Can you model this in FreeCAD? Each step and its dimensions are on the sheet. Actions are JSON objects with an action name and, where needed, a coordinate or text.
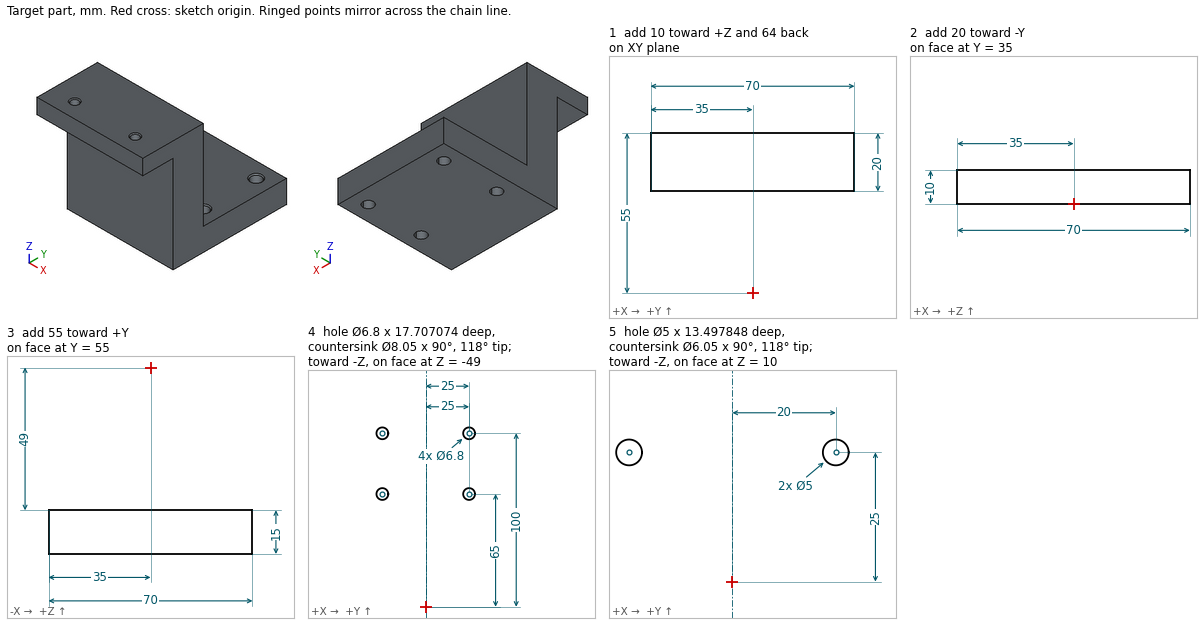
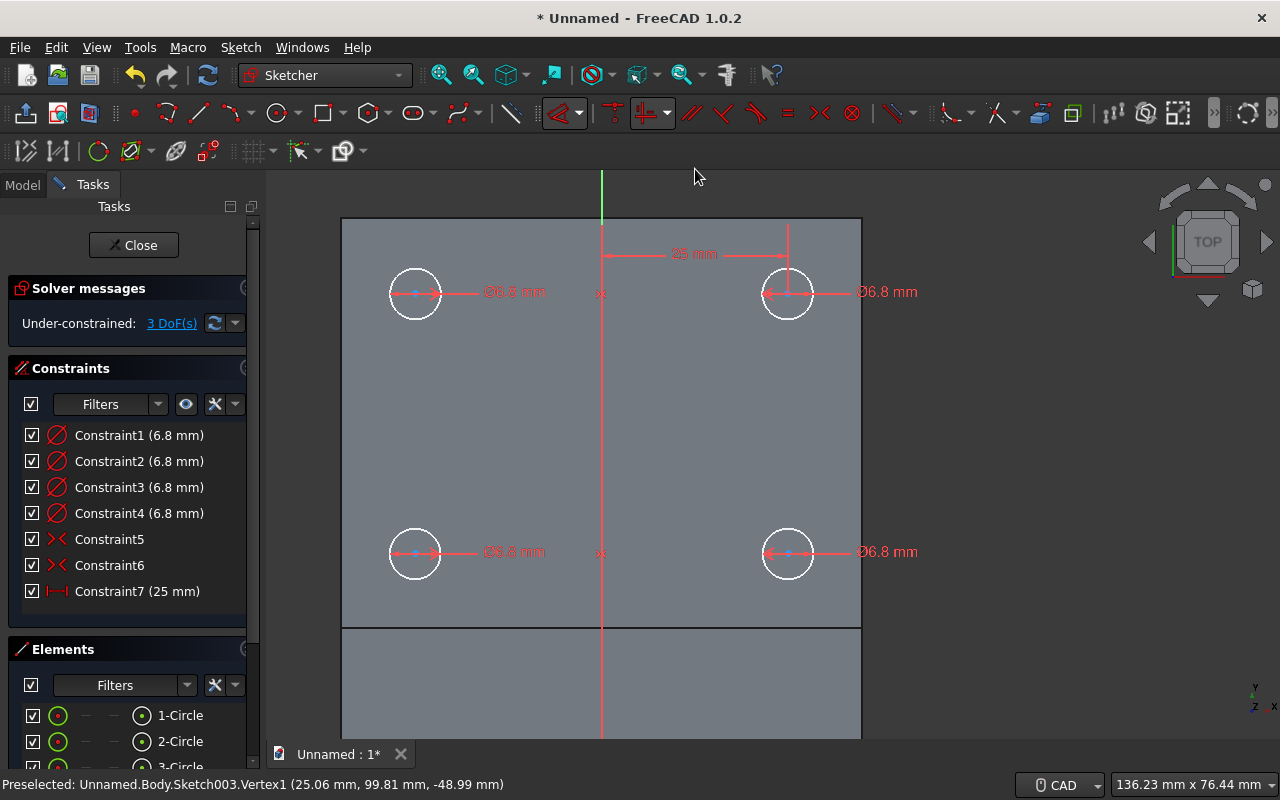
{"action": "left_click", "coordinate": [788, 554]}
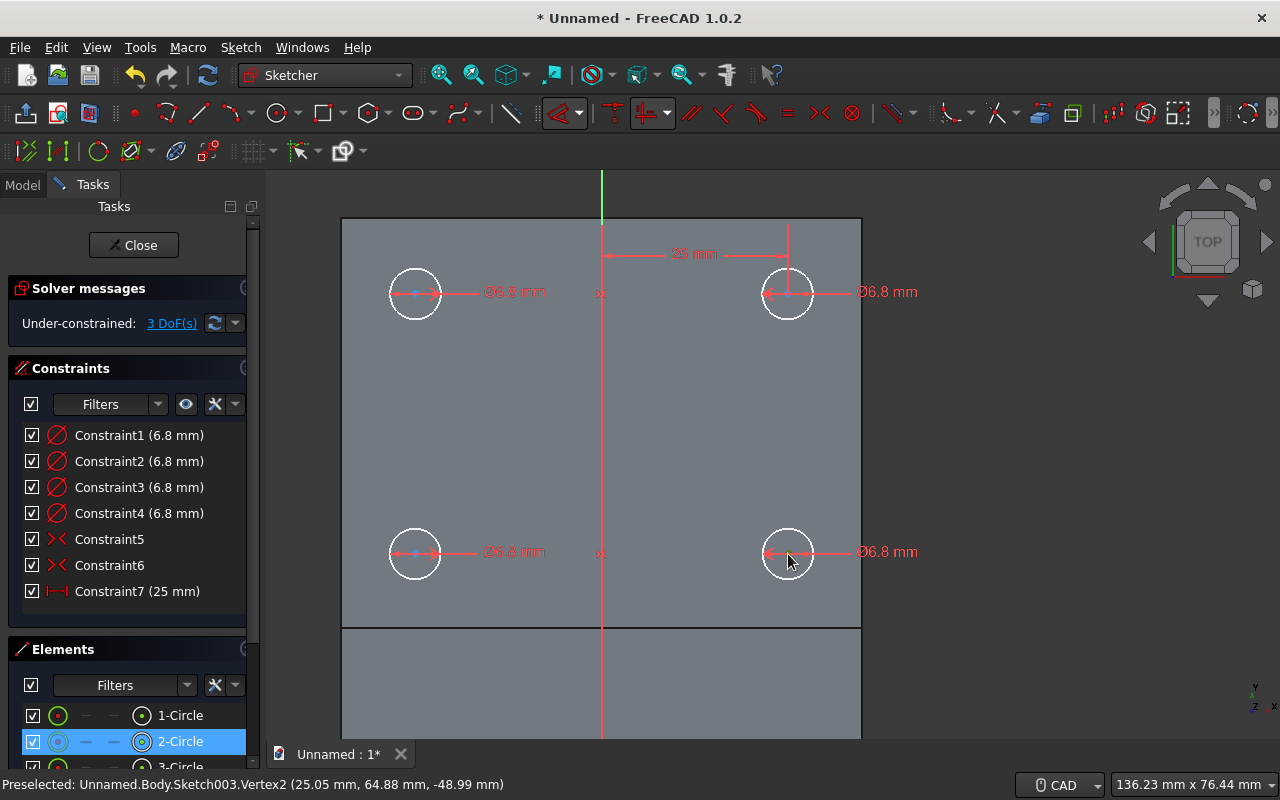
{"action": "key", "text": "l"}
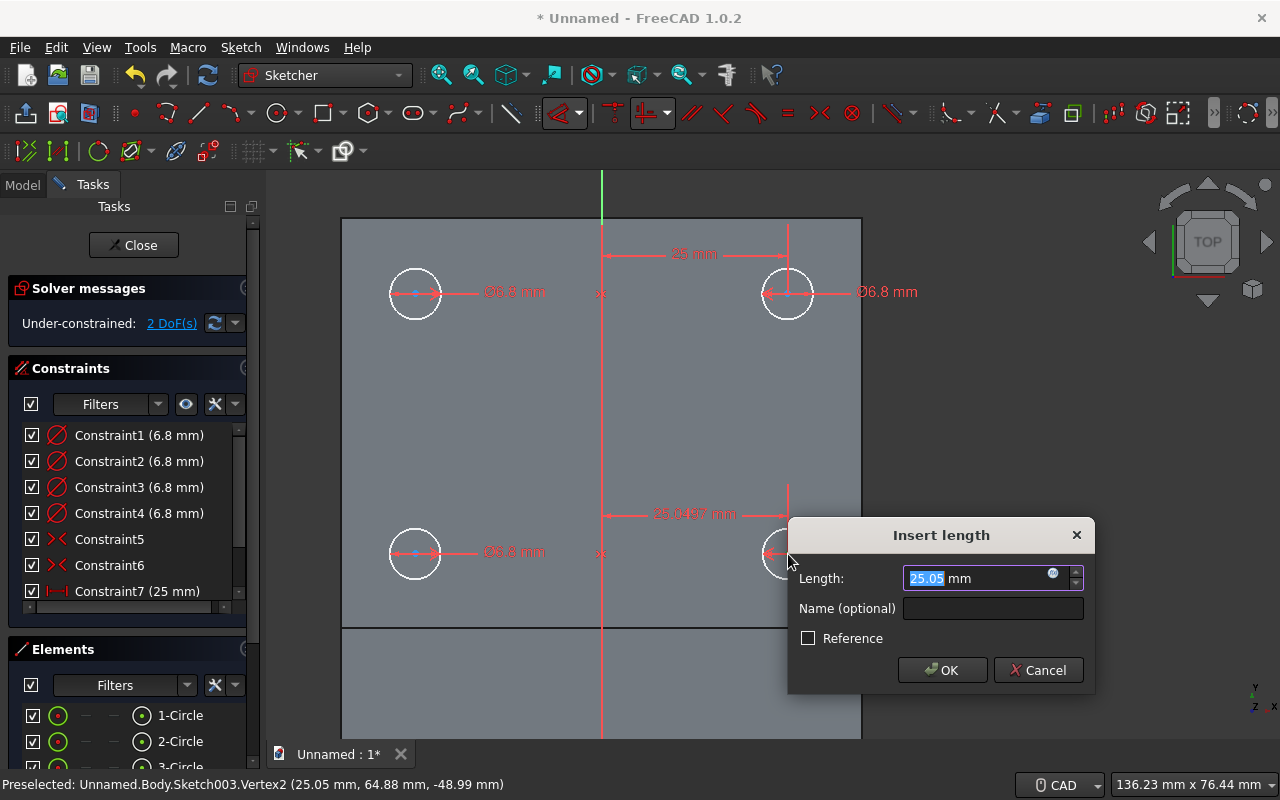
{"action": "type", "text": "25"}
{"action": "key", "text": "Return"}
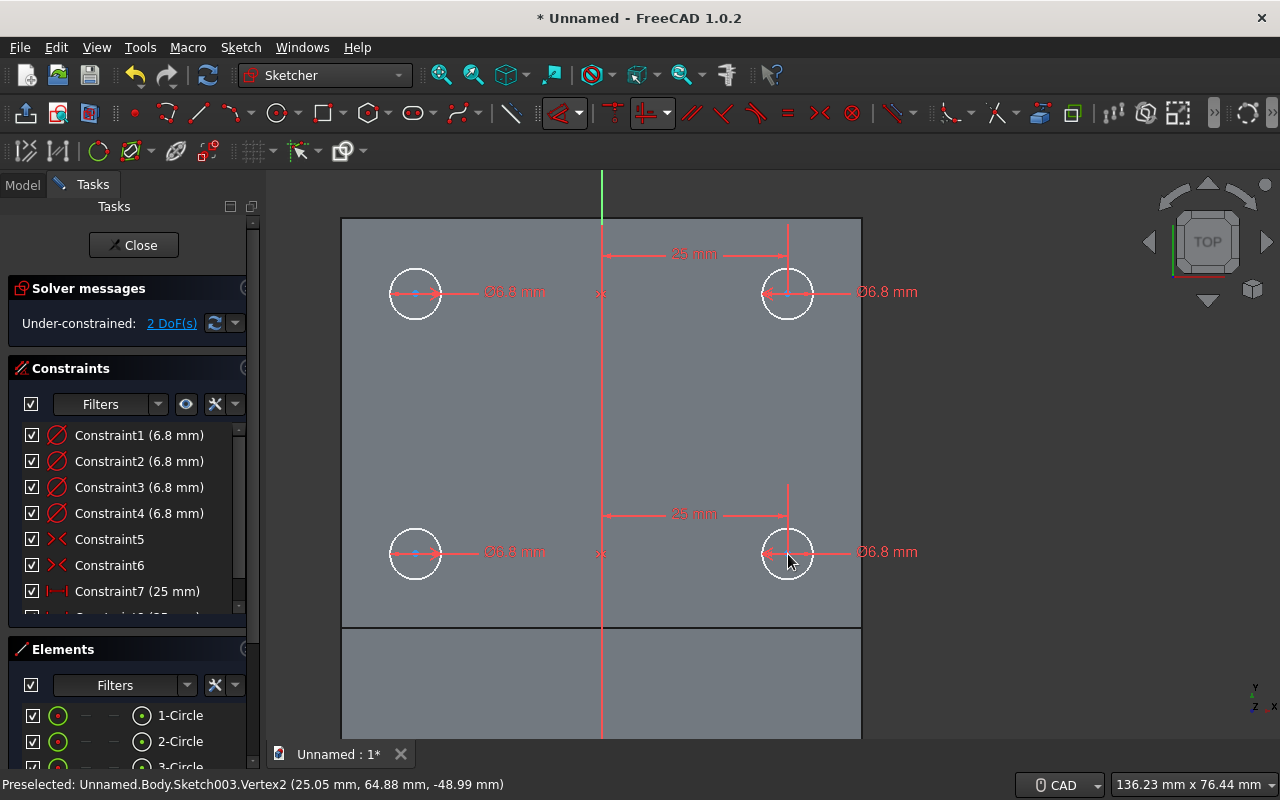
{"action": "left_click", "coordinate": [788, 554]}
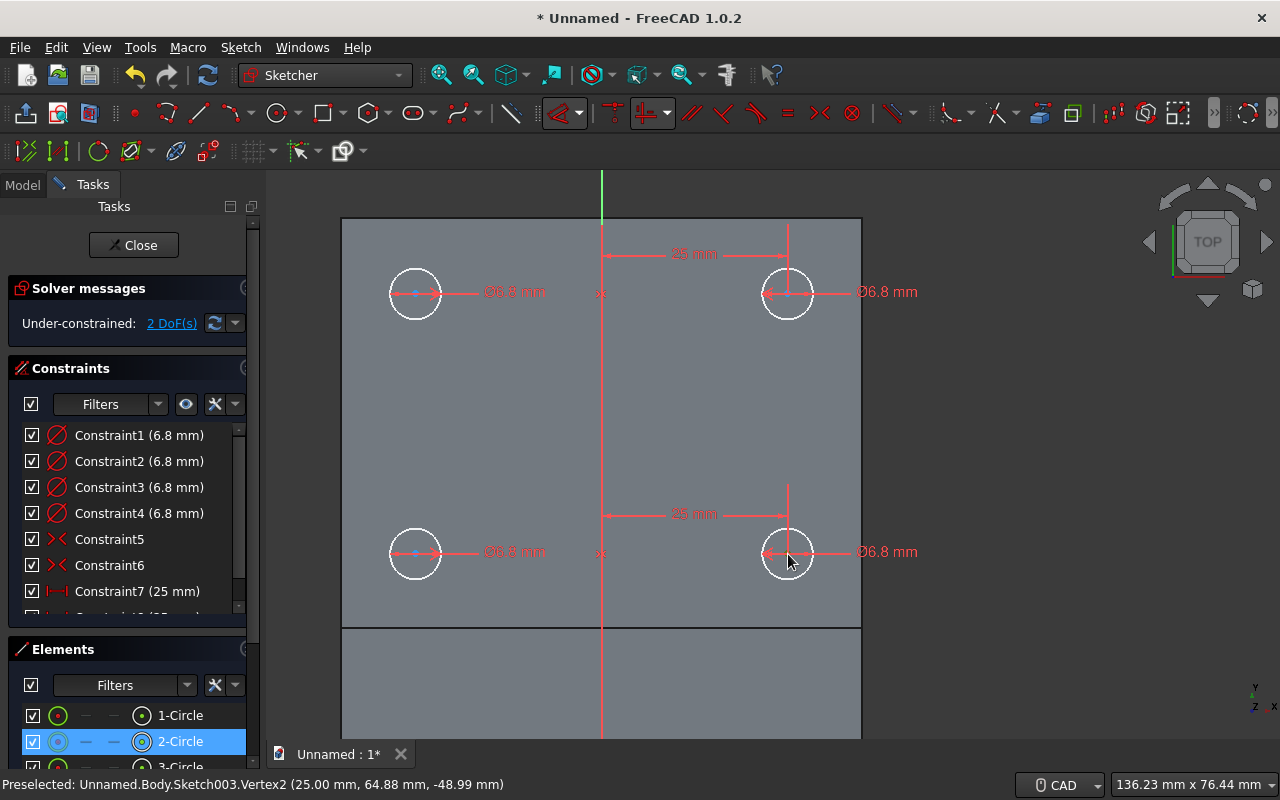
{"action": "key", "text": "i"}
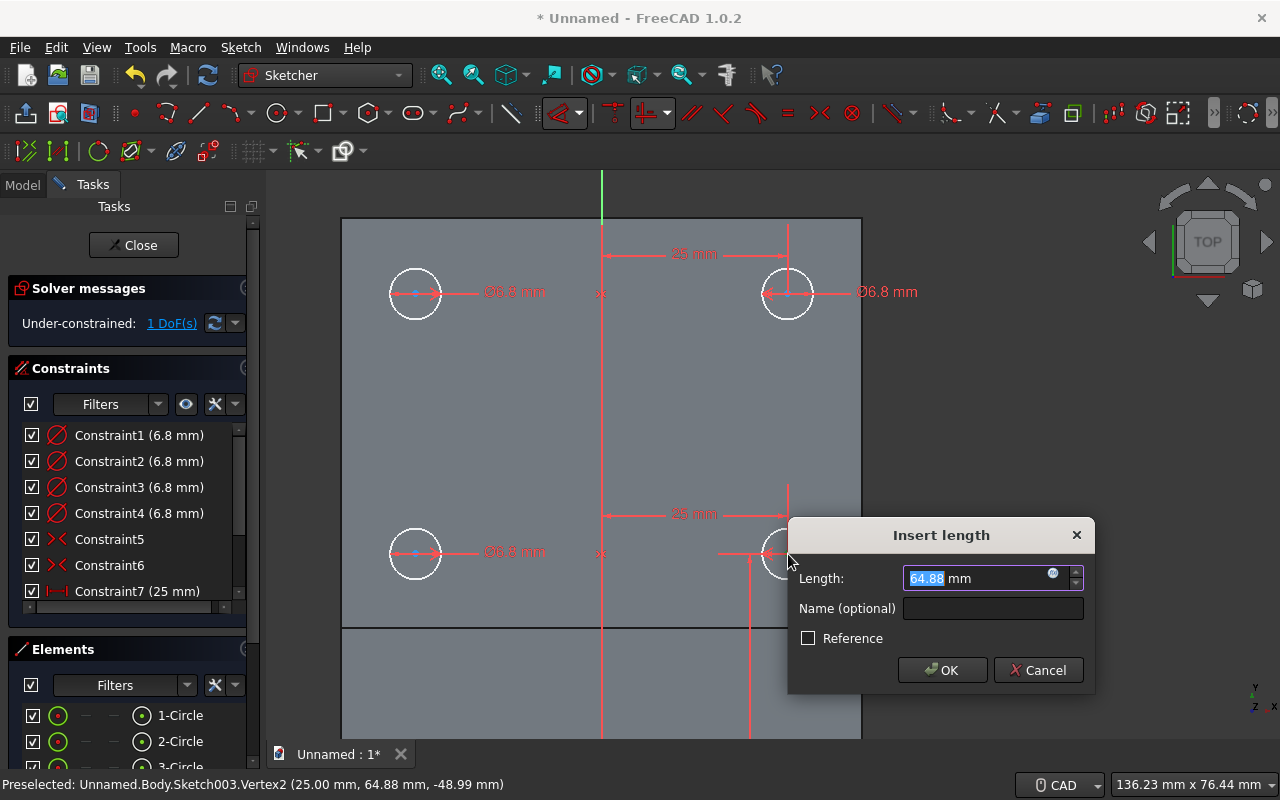
{"action": "type", "text": "65"}
{"action": "key", "text": "Return"}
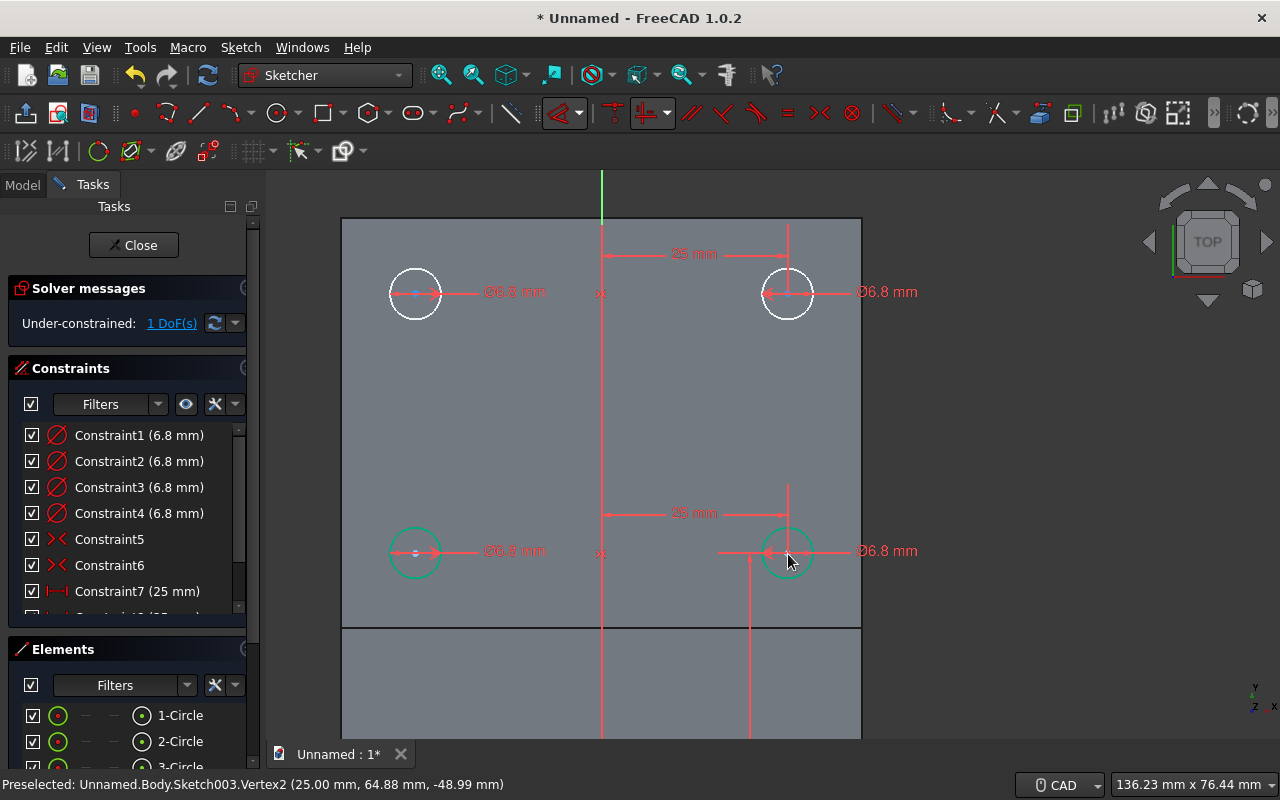
{"action": "left_click", "coordinate": [788, 294]}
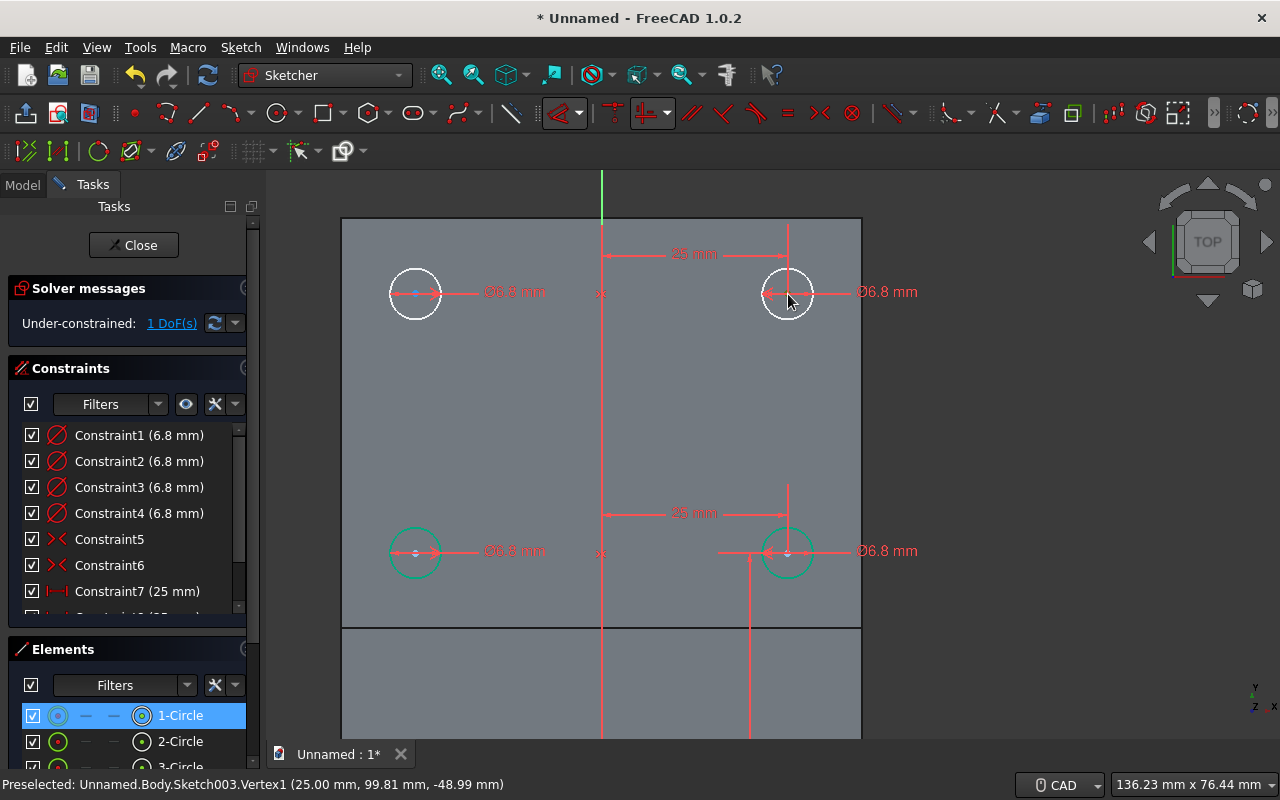
{"action": "left_click", "coordinate": [582, 114]}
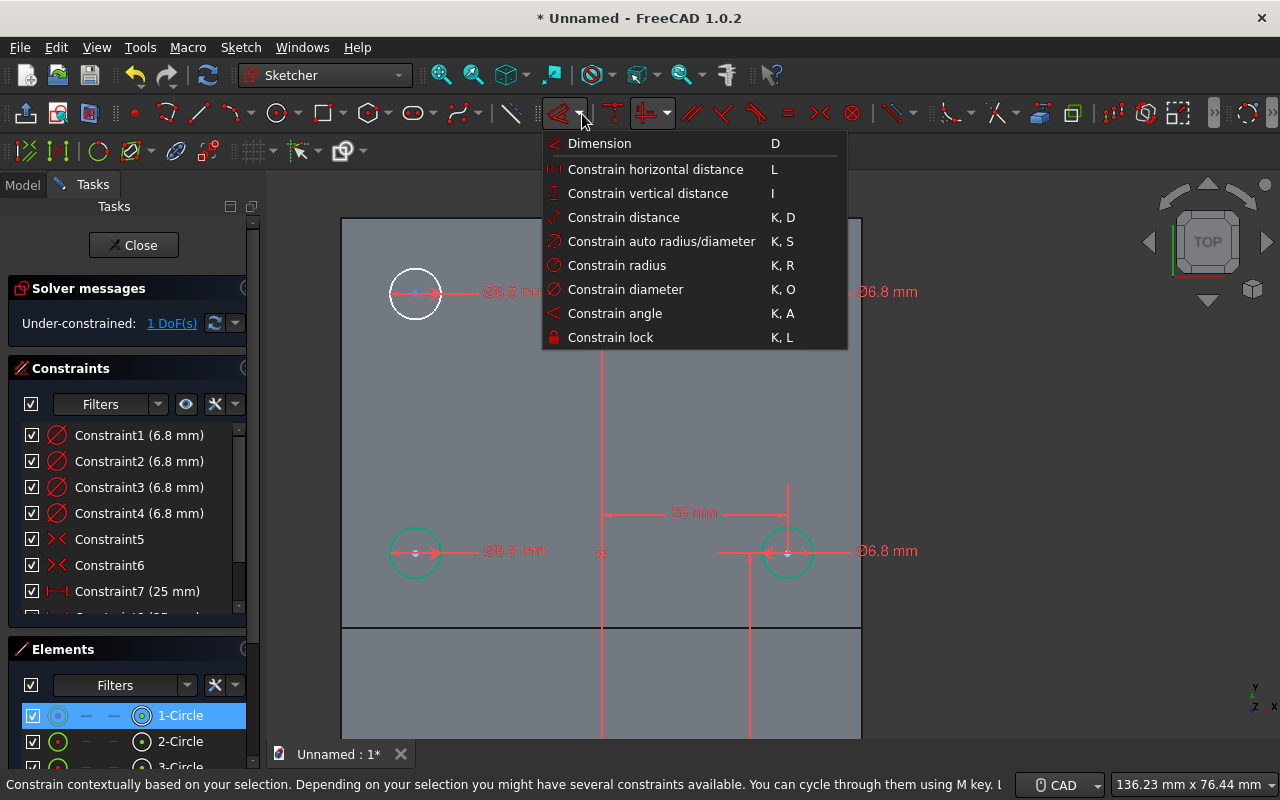
{"action": "left_click", "coordinate": [695, 193]}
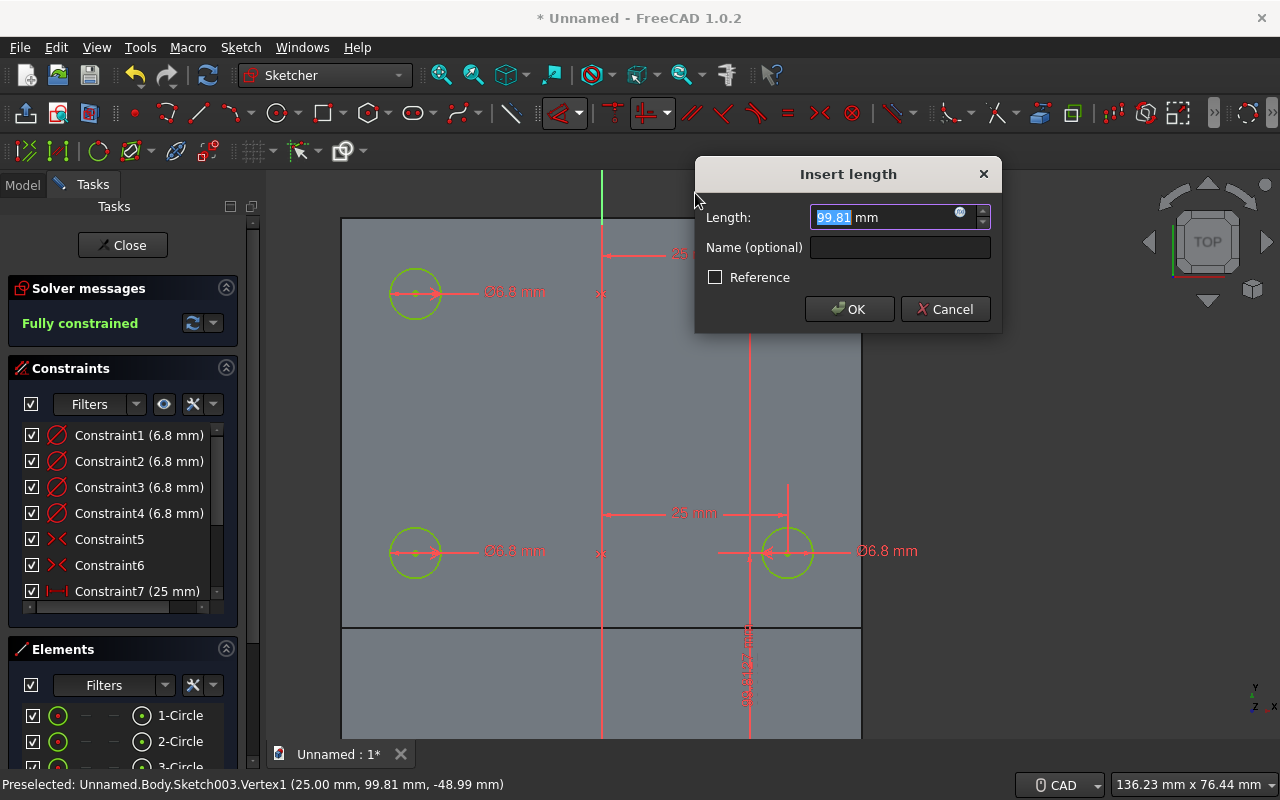
{"action": "type", "text": "100"}
{"action": "key", "text": "Return"}